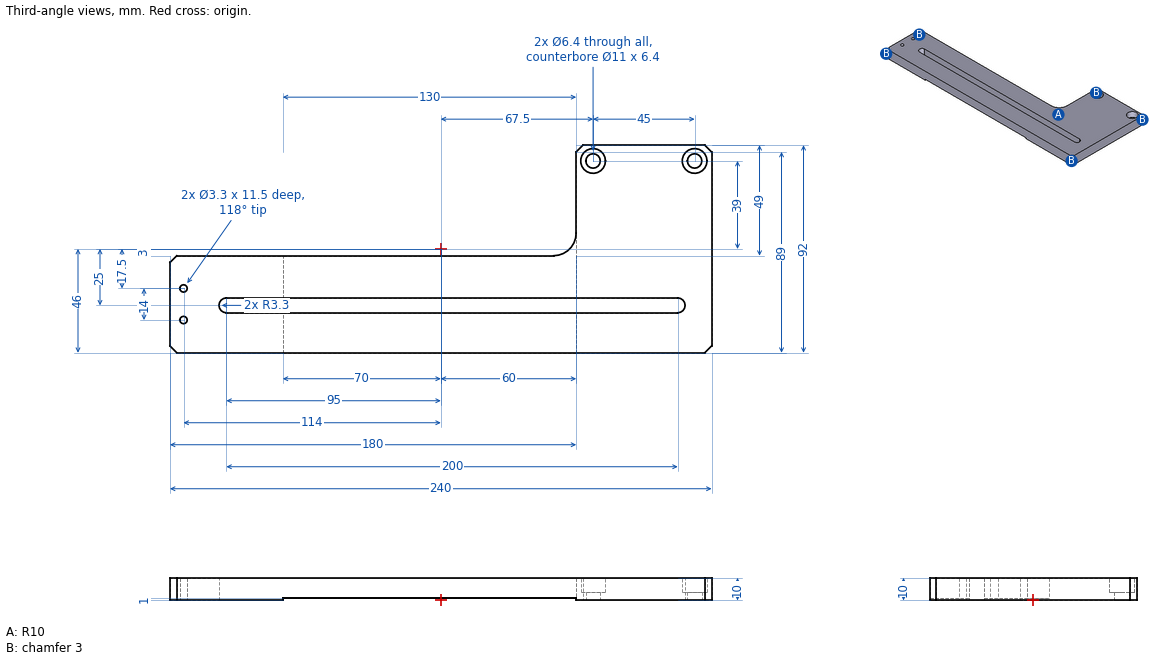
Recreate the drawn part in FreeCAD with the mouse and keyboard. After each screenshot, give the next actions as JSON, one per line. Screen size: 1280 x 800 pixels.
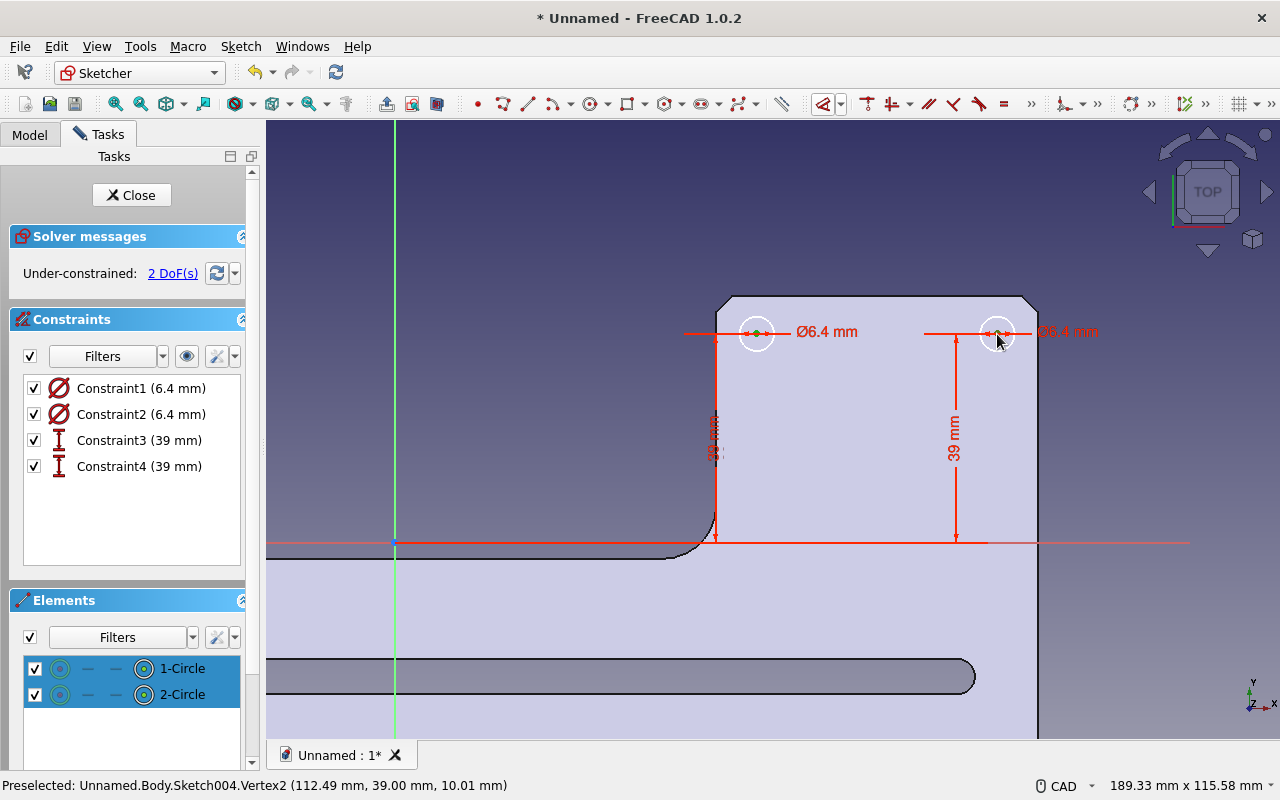
{"action": "key", "text": "l"}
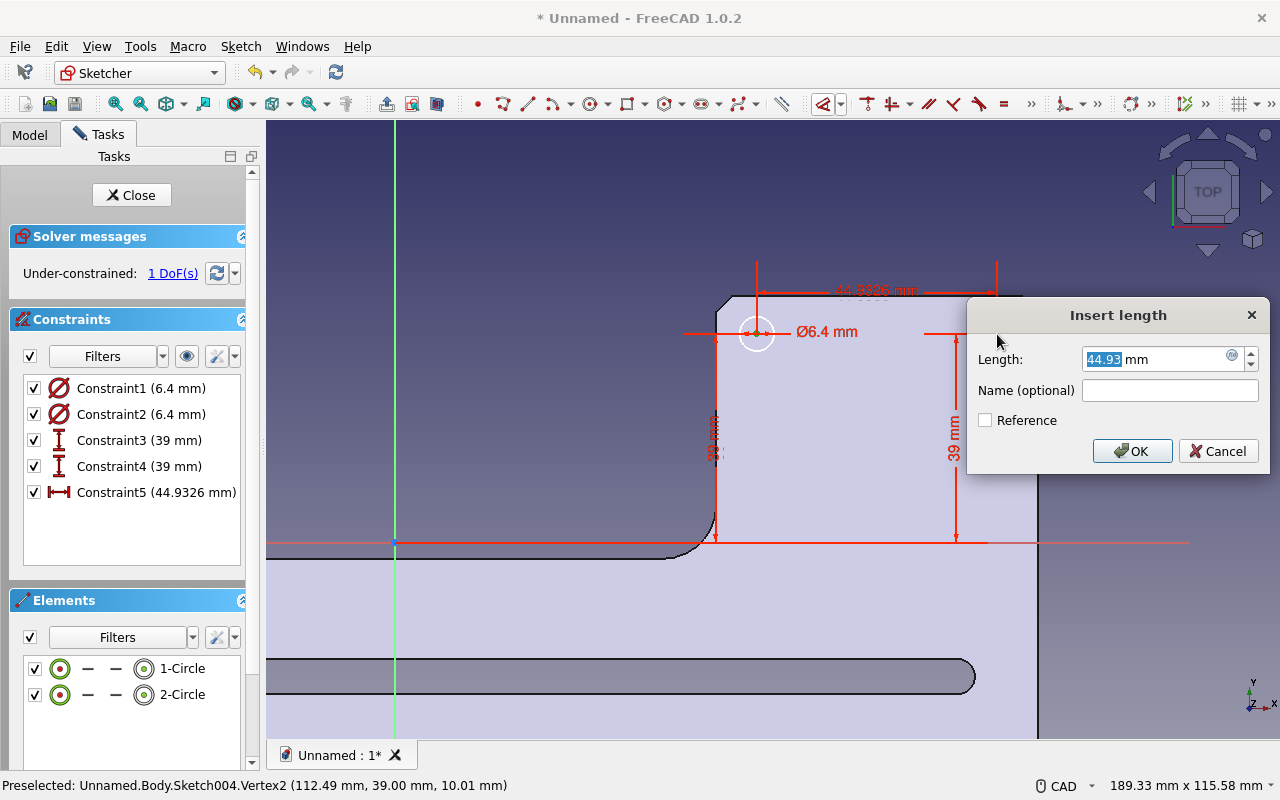
{"action": "type", "text": "45"}
{"action": "key", "text": "Return"}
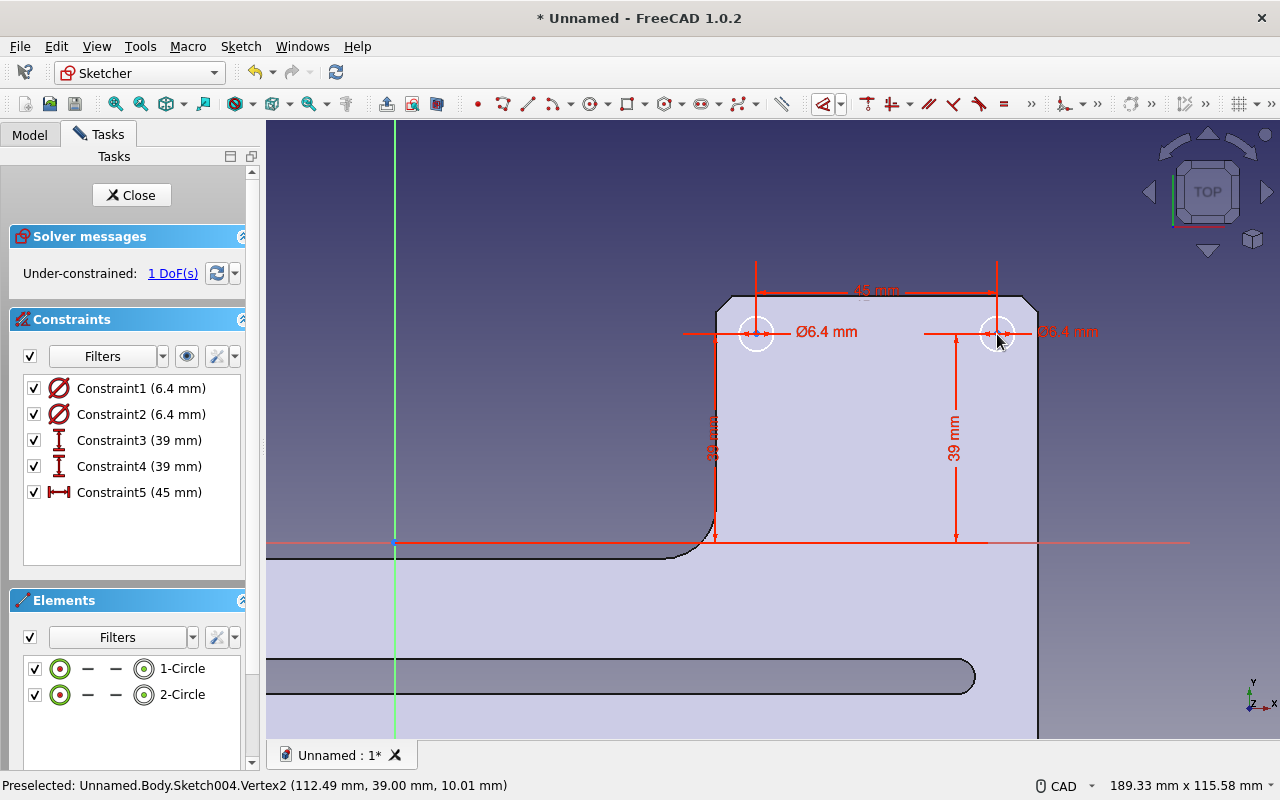
{"action": "left_click", "coordinate": [756, 334]}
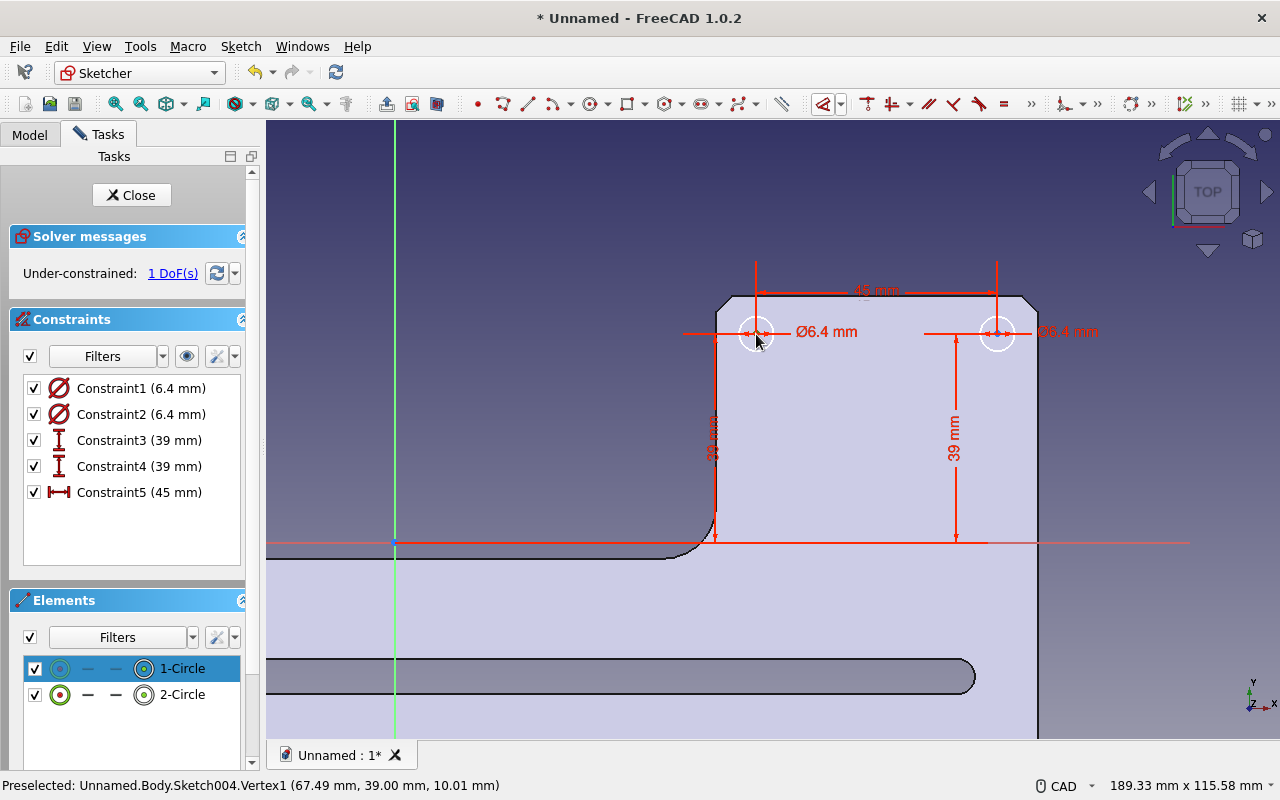
{"action": "key", "text": "l"}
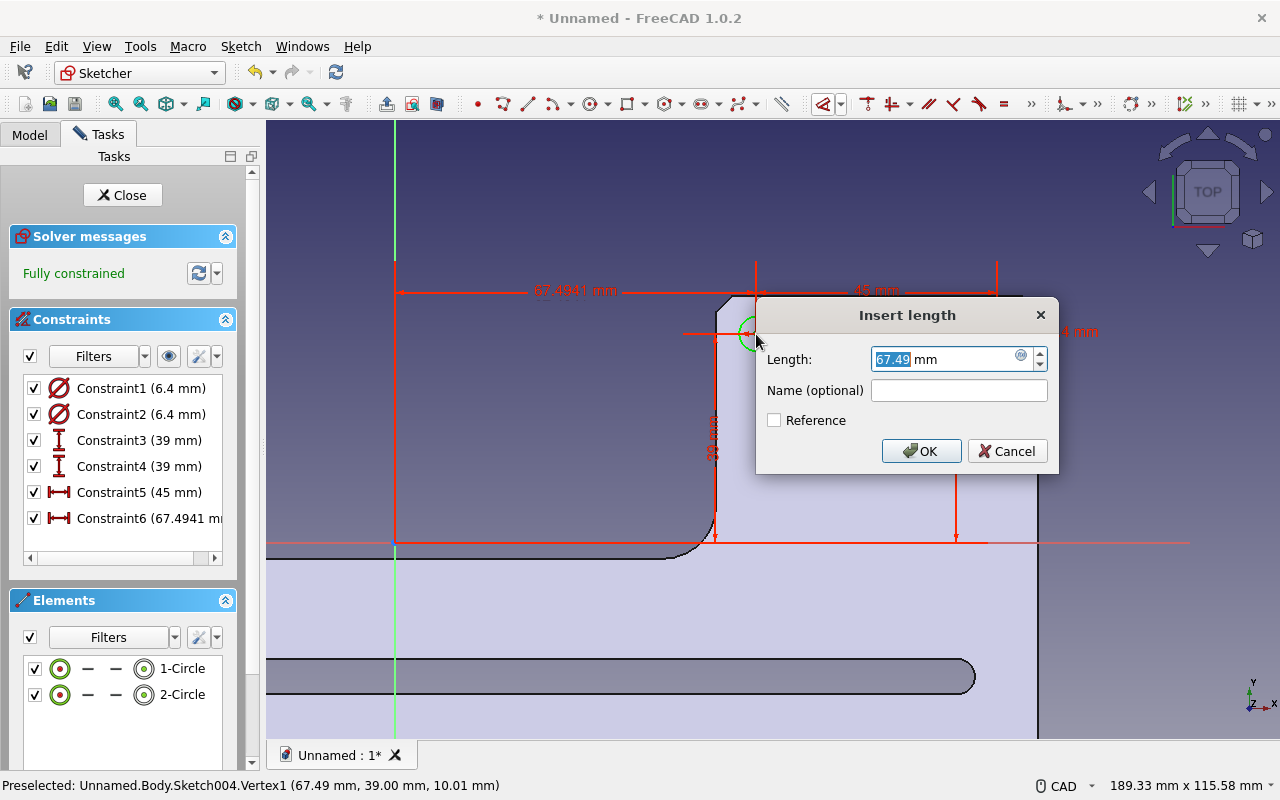
{"action": "type", "text": "67.5"}
{"action": "key", "text": "Return"}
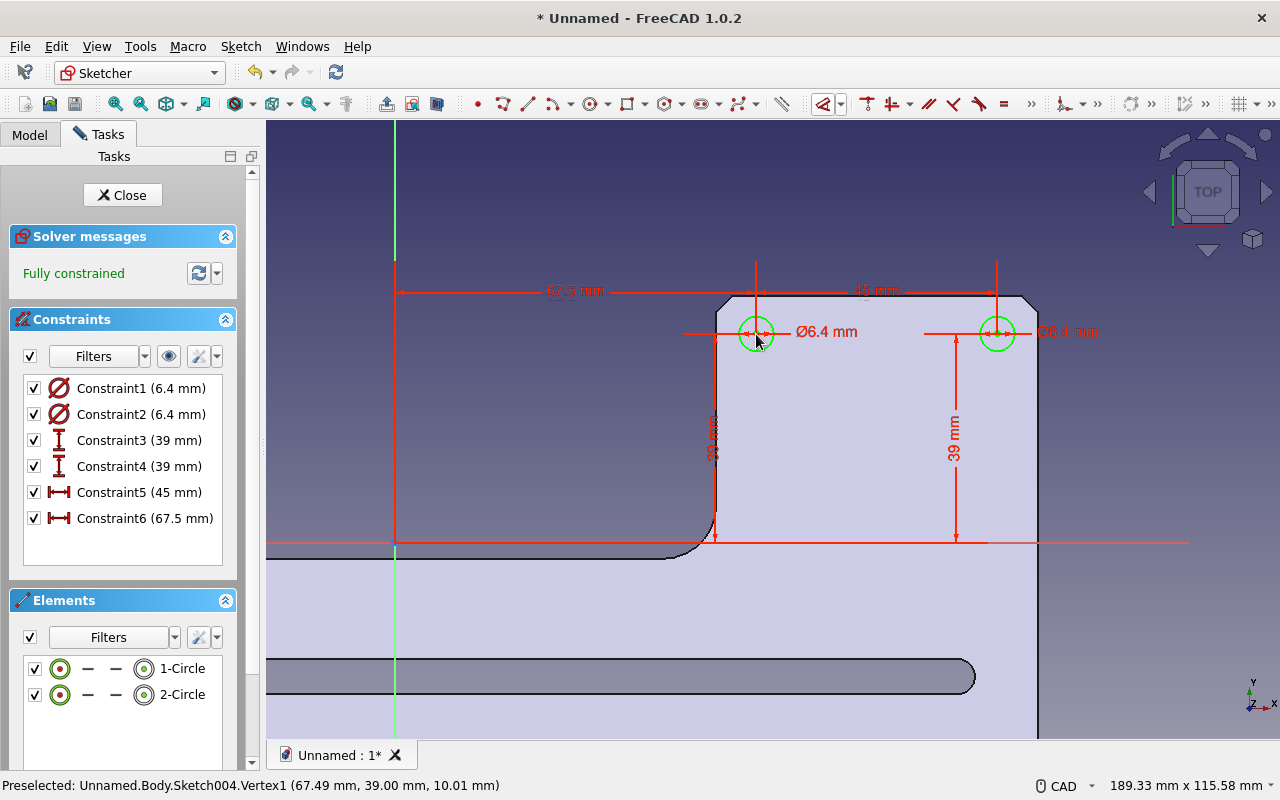
{"action": "left_click", "coordinate": [123, 195]}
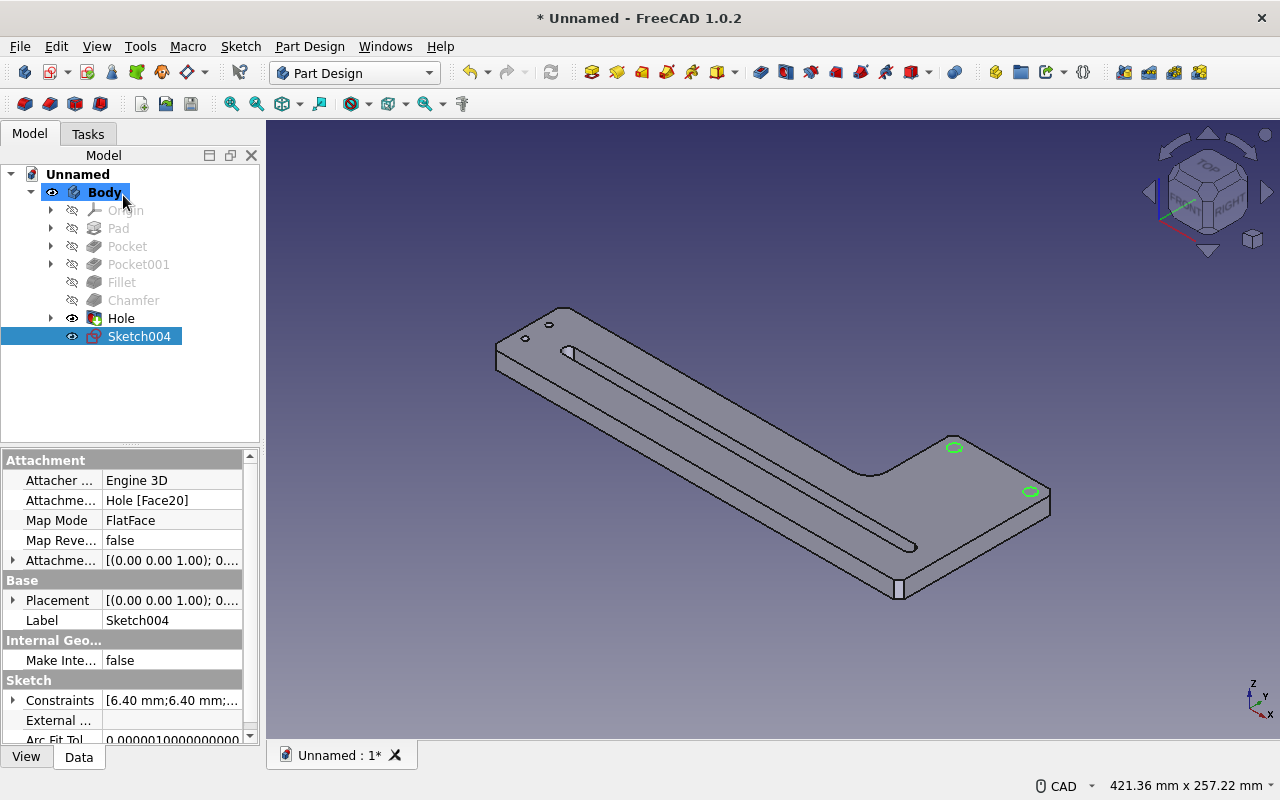
{"action": "left_click", "coordinate": [786, 72]}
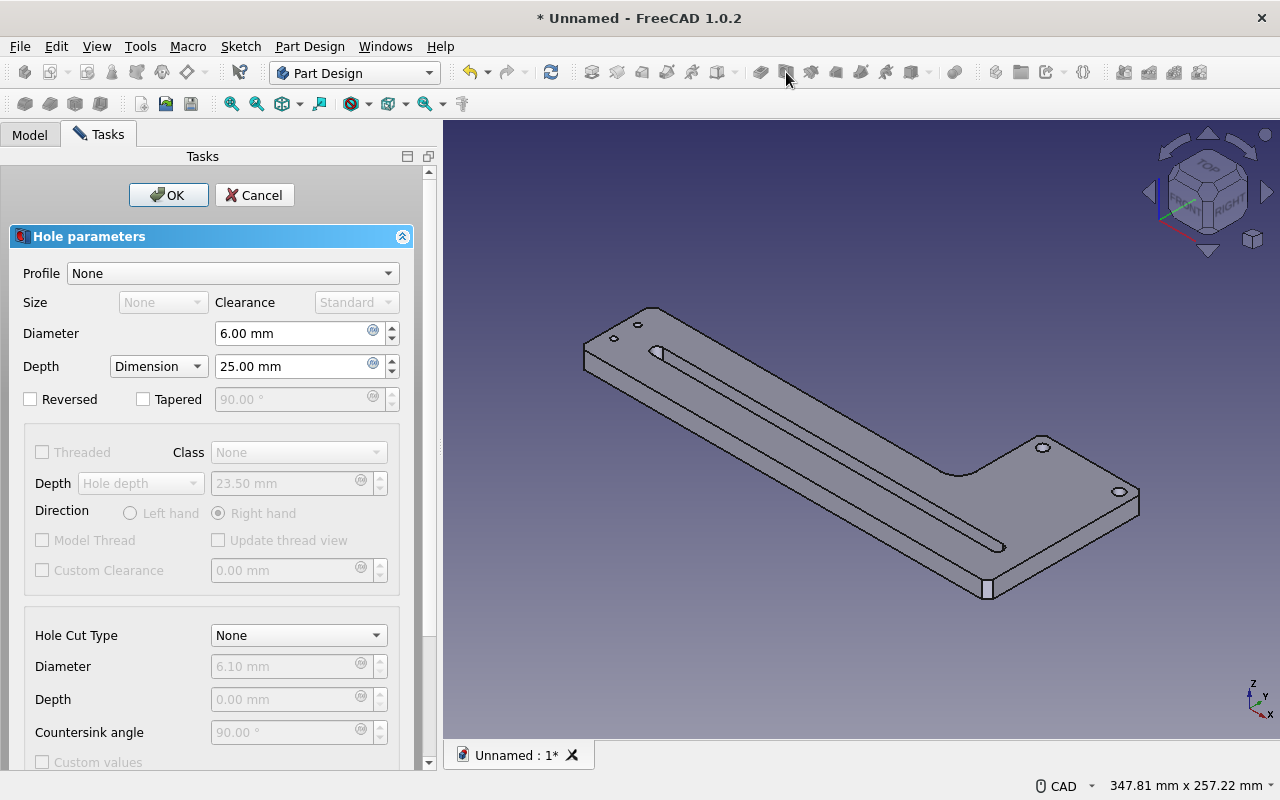
{"action": "triple_click", "coordinate": [300, 334]}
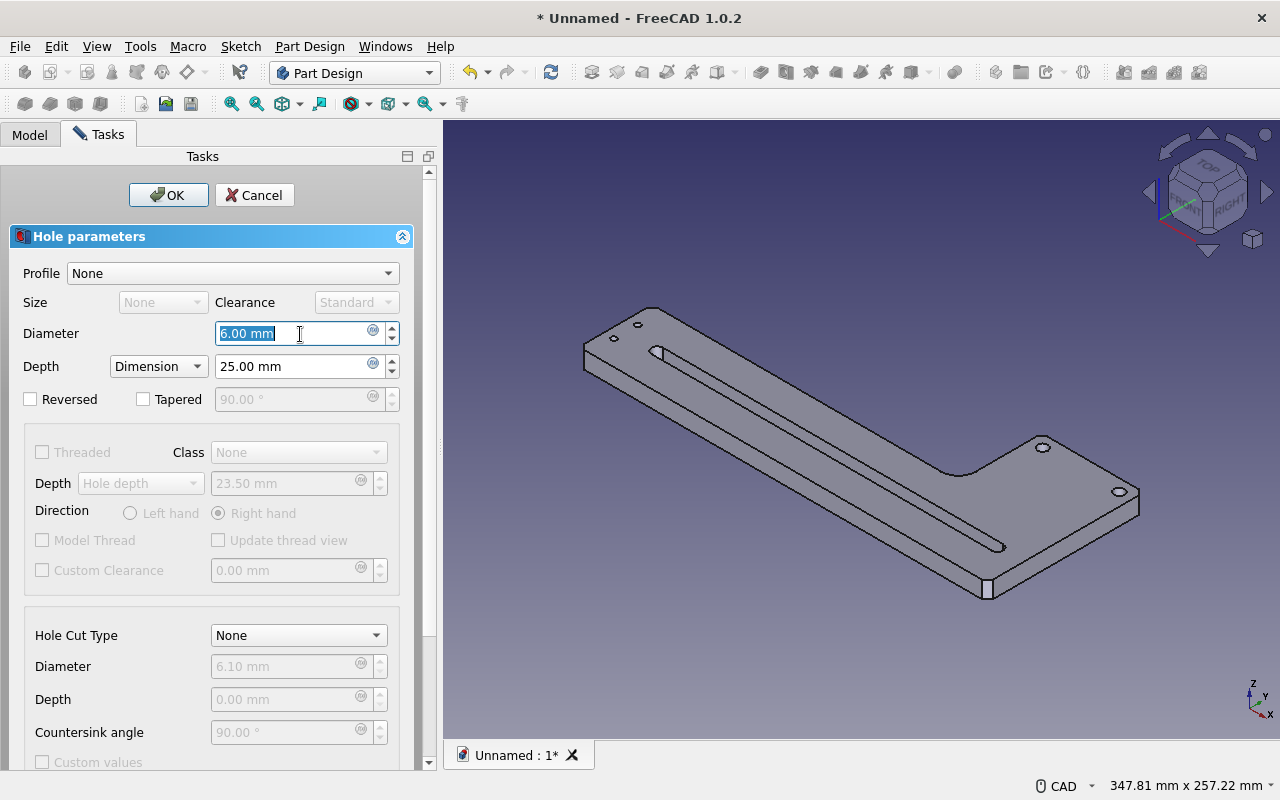
{"action": "type", "text": "6.4"}
{"action": "key", "text": "Tab"}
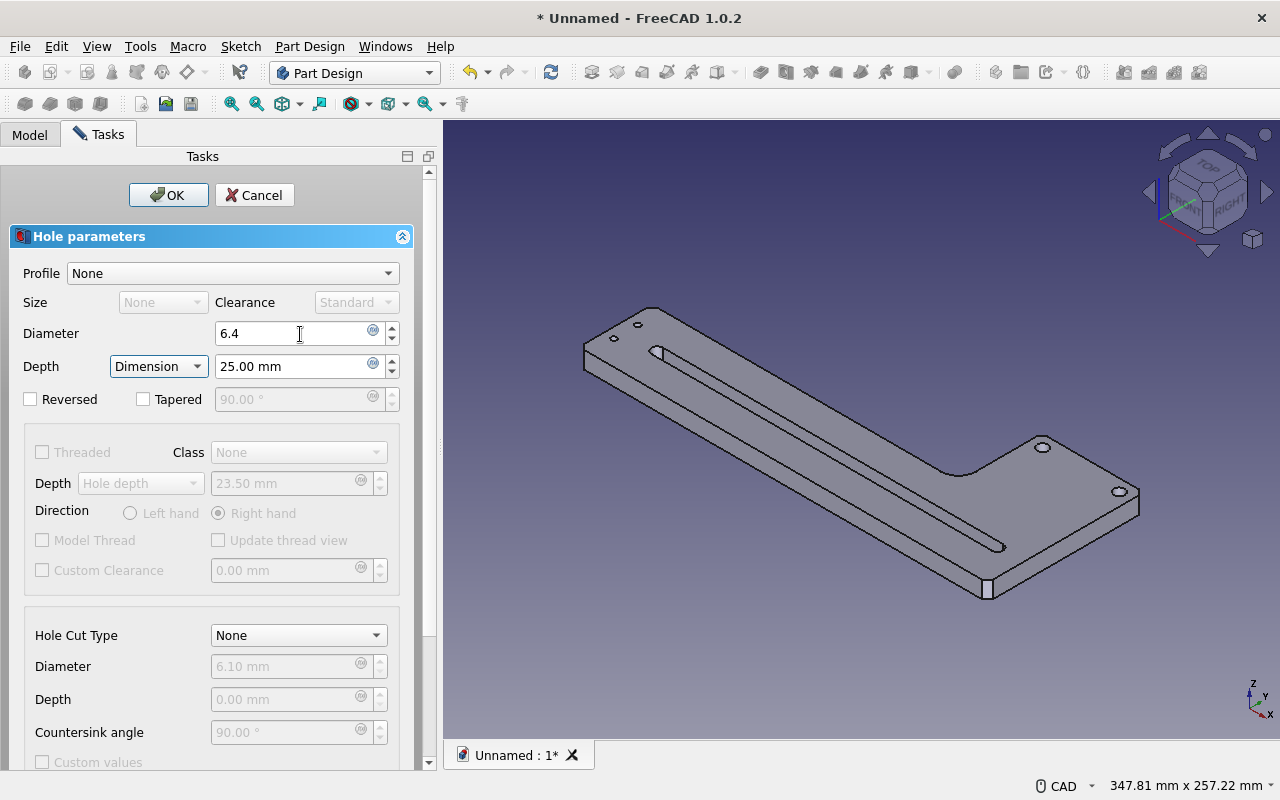
{"action": "left_click", "coordinate": [160, 366]}